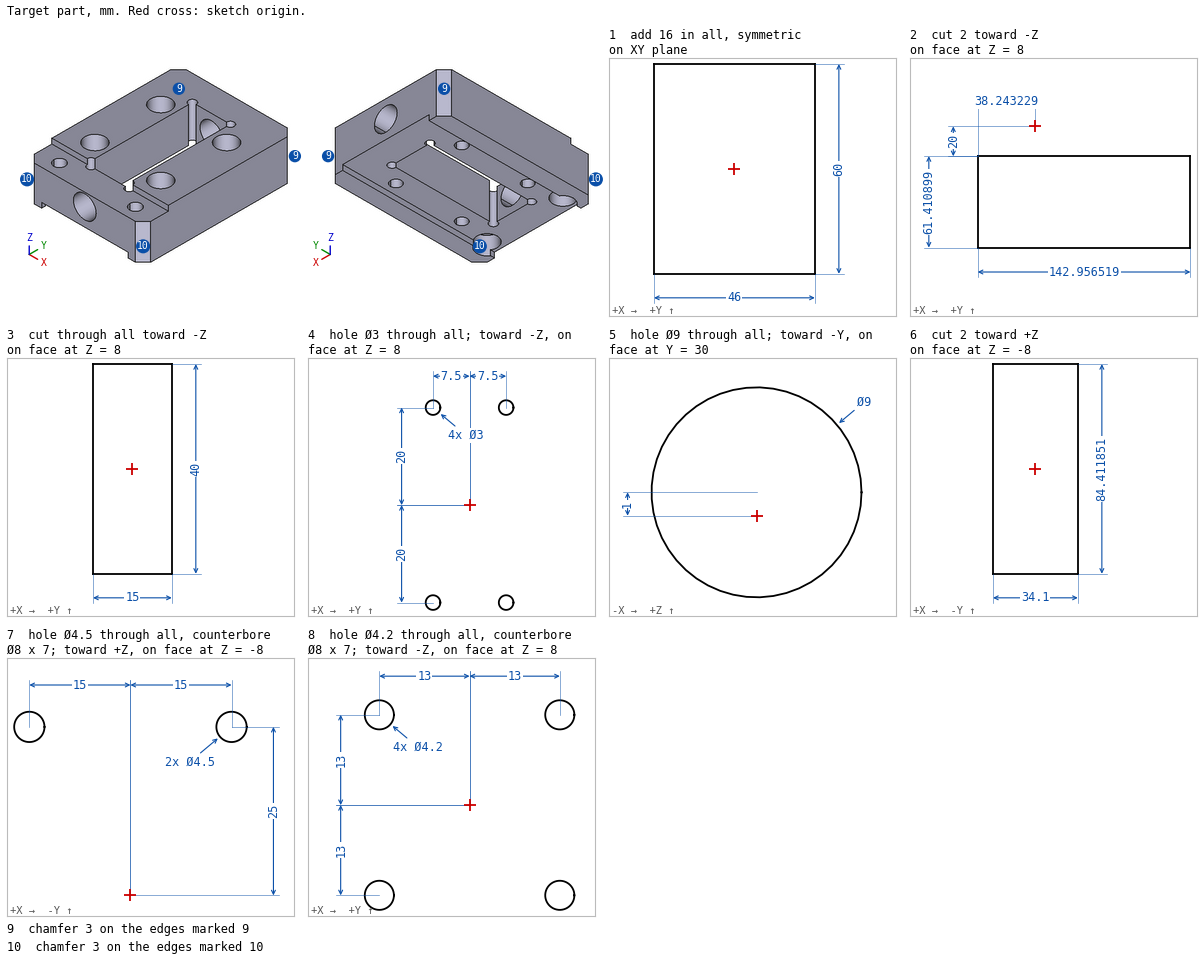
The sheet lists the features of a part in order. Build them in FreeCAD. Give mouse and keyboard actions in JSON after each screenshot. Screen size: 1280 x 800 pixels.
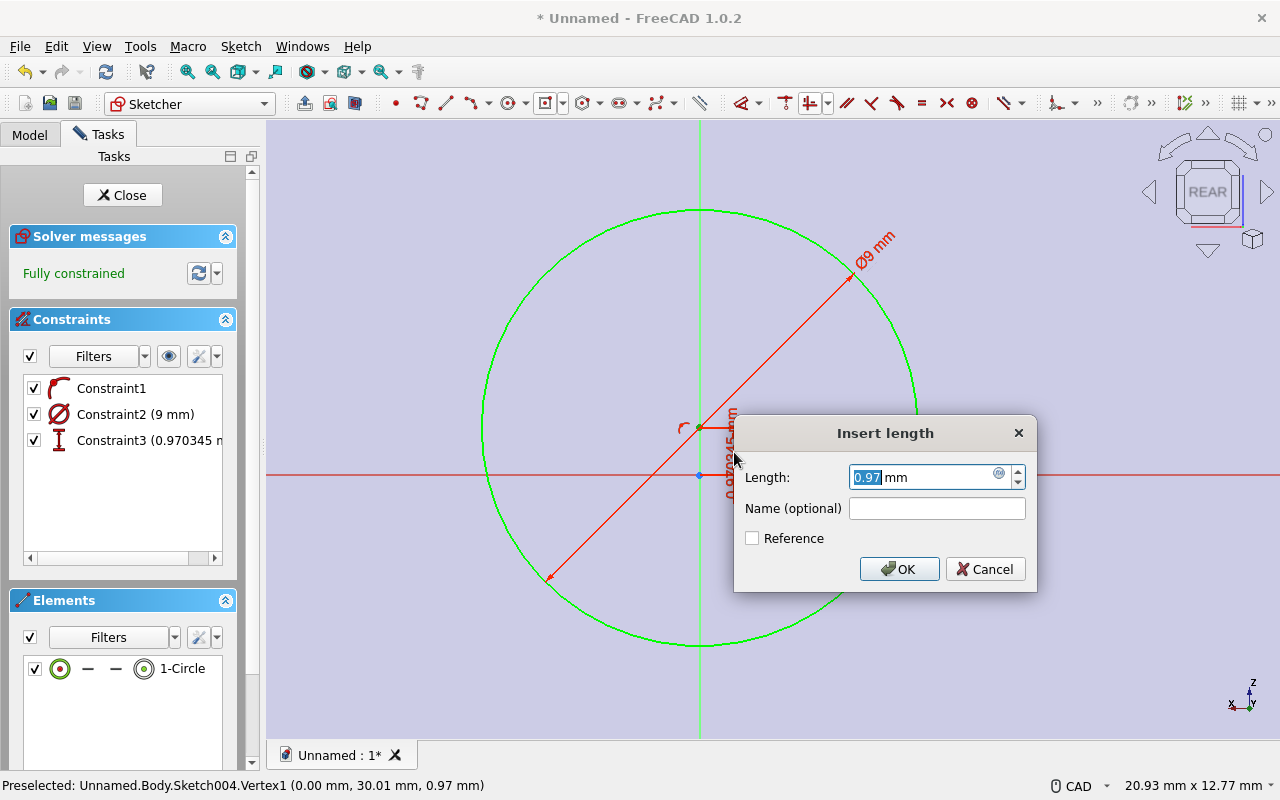
{"action": "type", "text": "1"}
{"action": "key", "text": "Return"}
{"action": "key", "text": "Escape"}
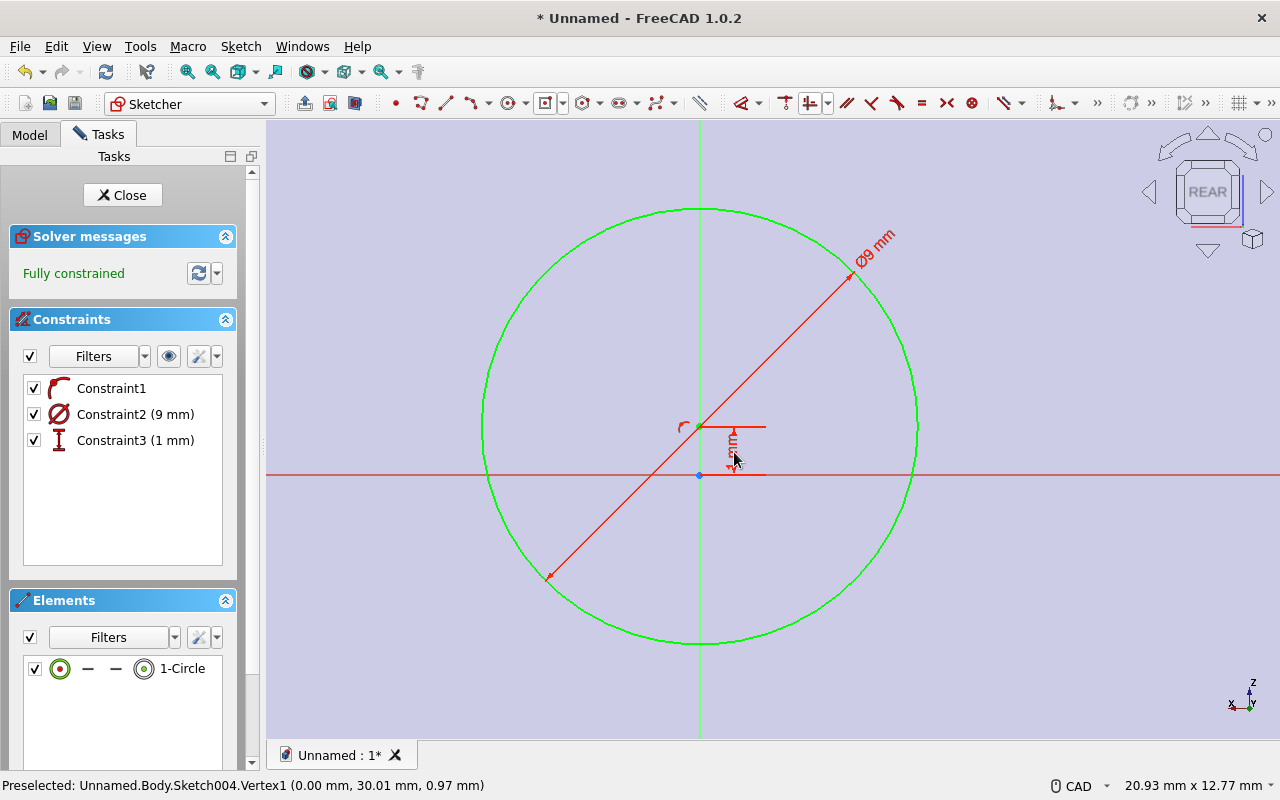
{"action": "left_click", "coordinate": [123, 195]}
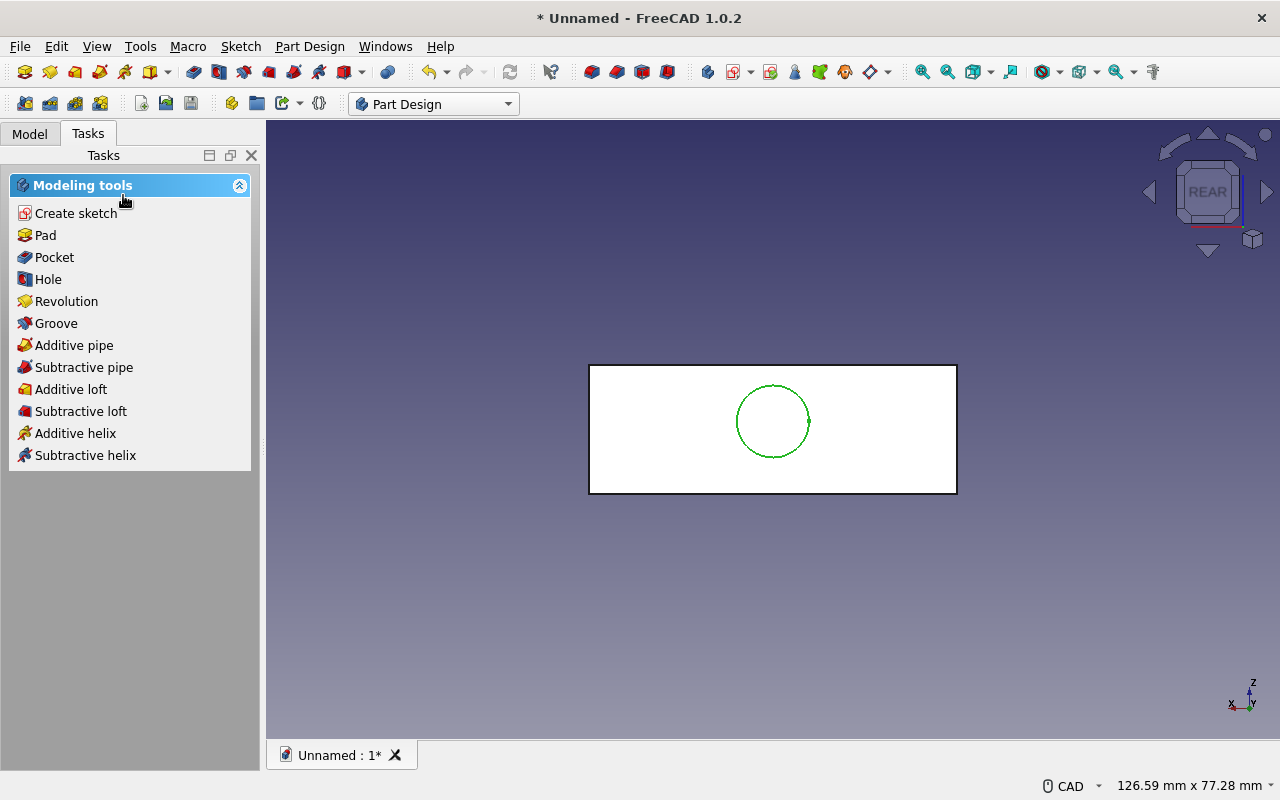
{"action": "left_click", "coordinate": [219, 72]}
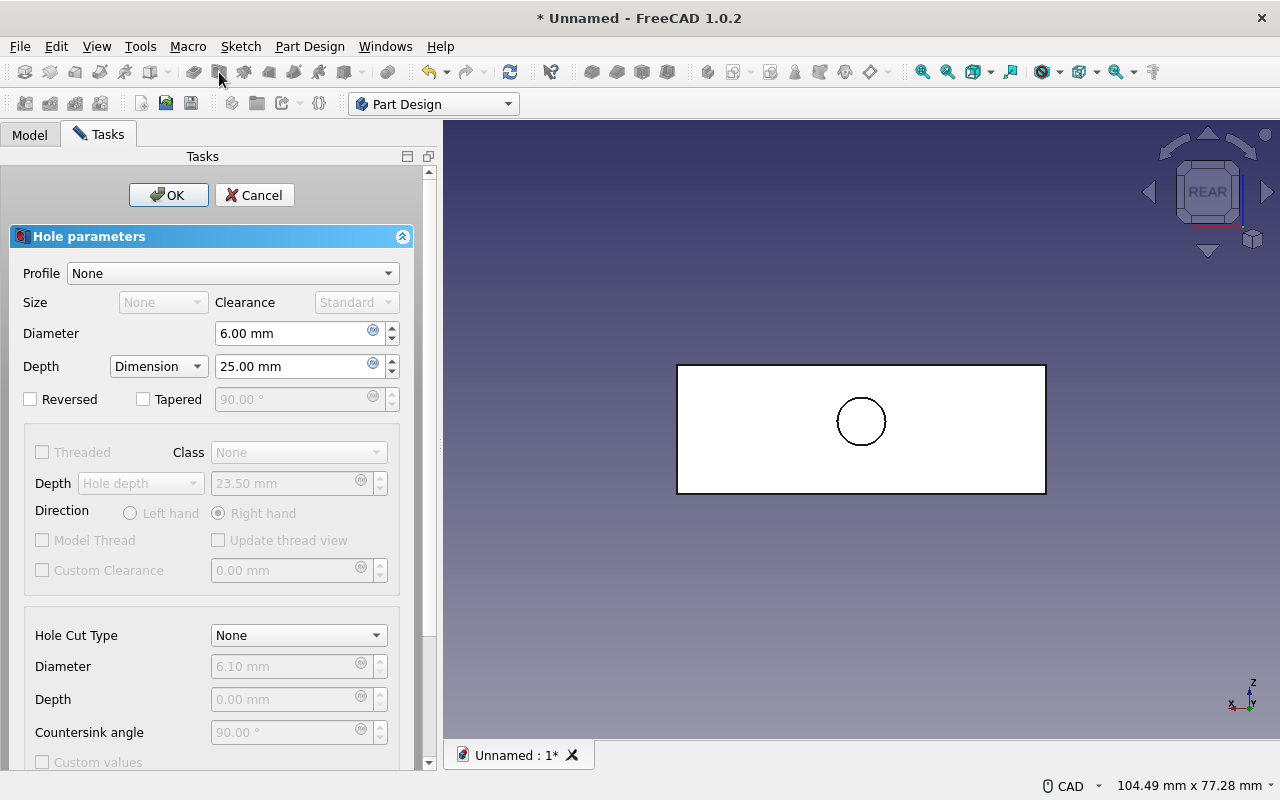
{"action": "triple_click", "coordinate": [300, 334]}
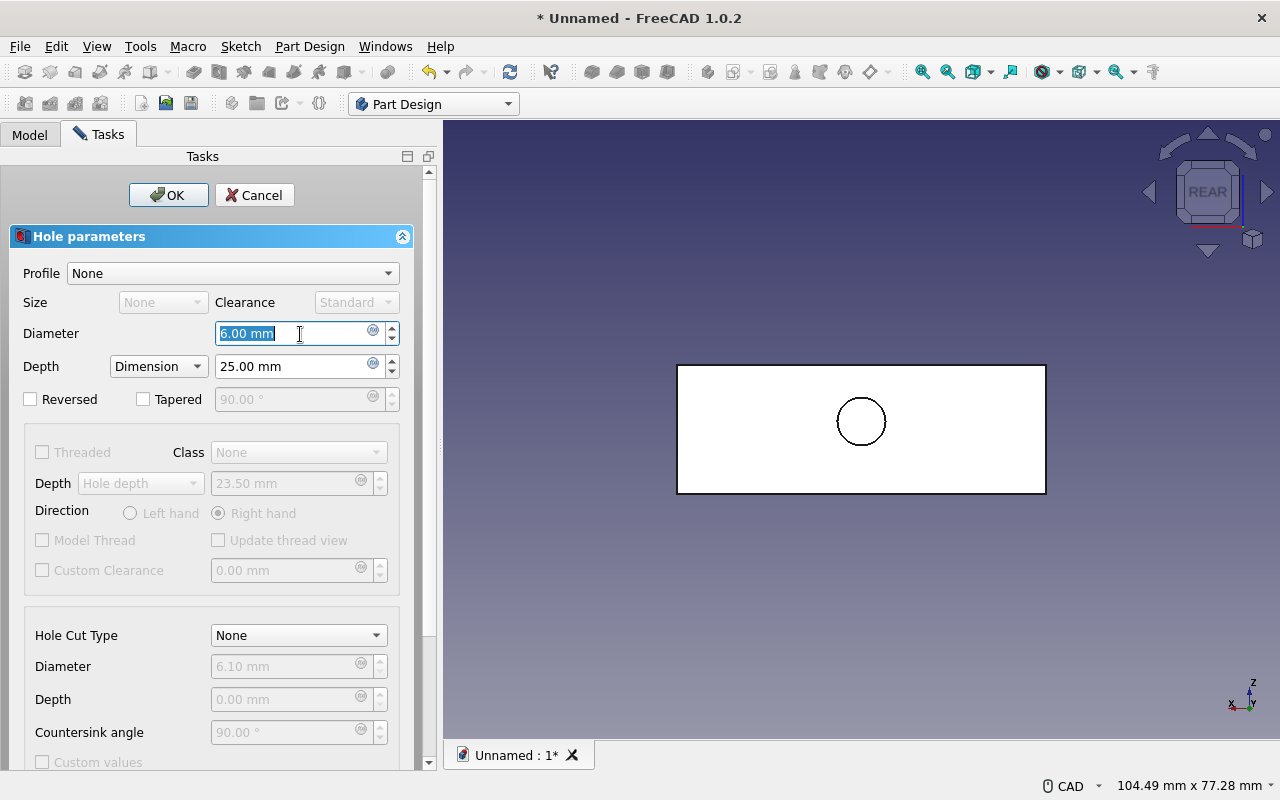
{"action": "type", "text": "9"}
{"action": "key", "text": "Tab"}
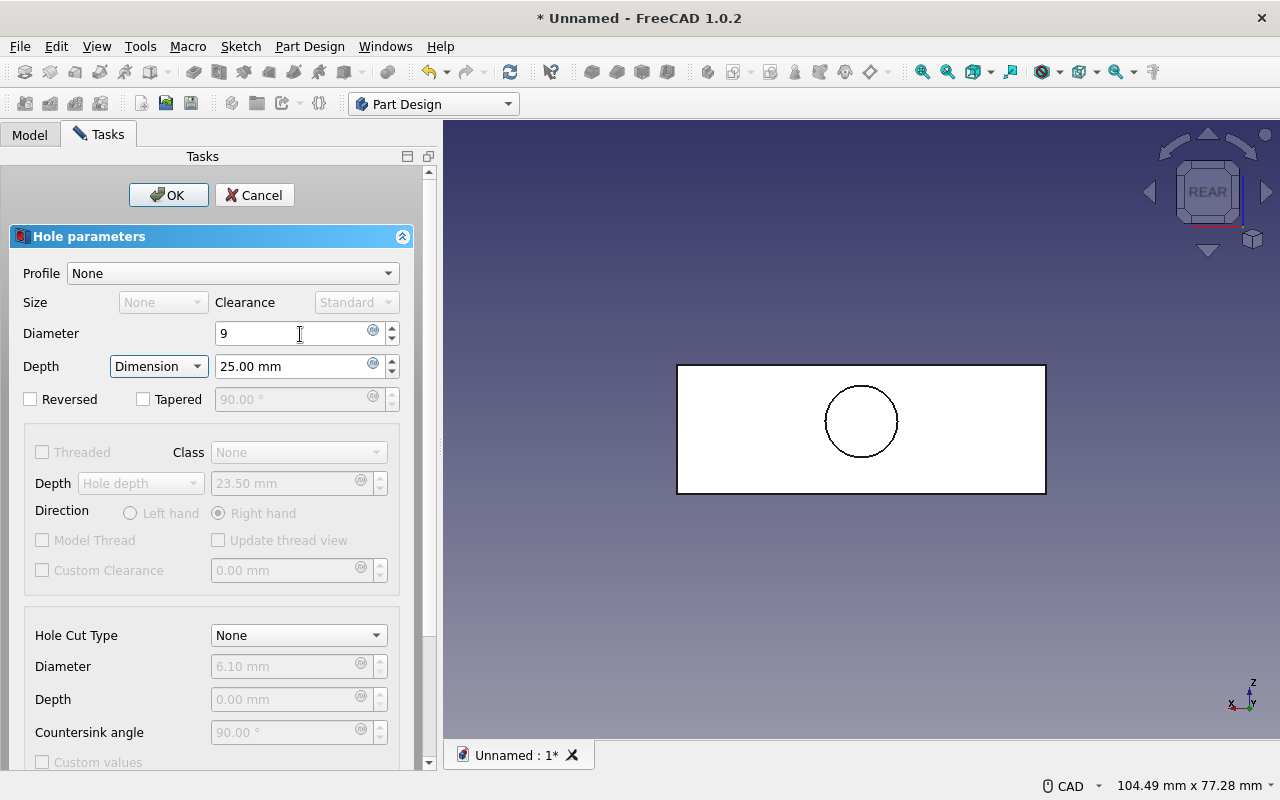
{"action": "left_click", "coordinate": [160, 366]}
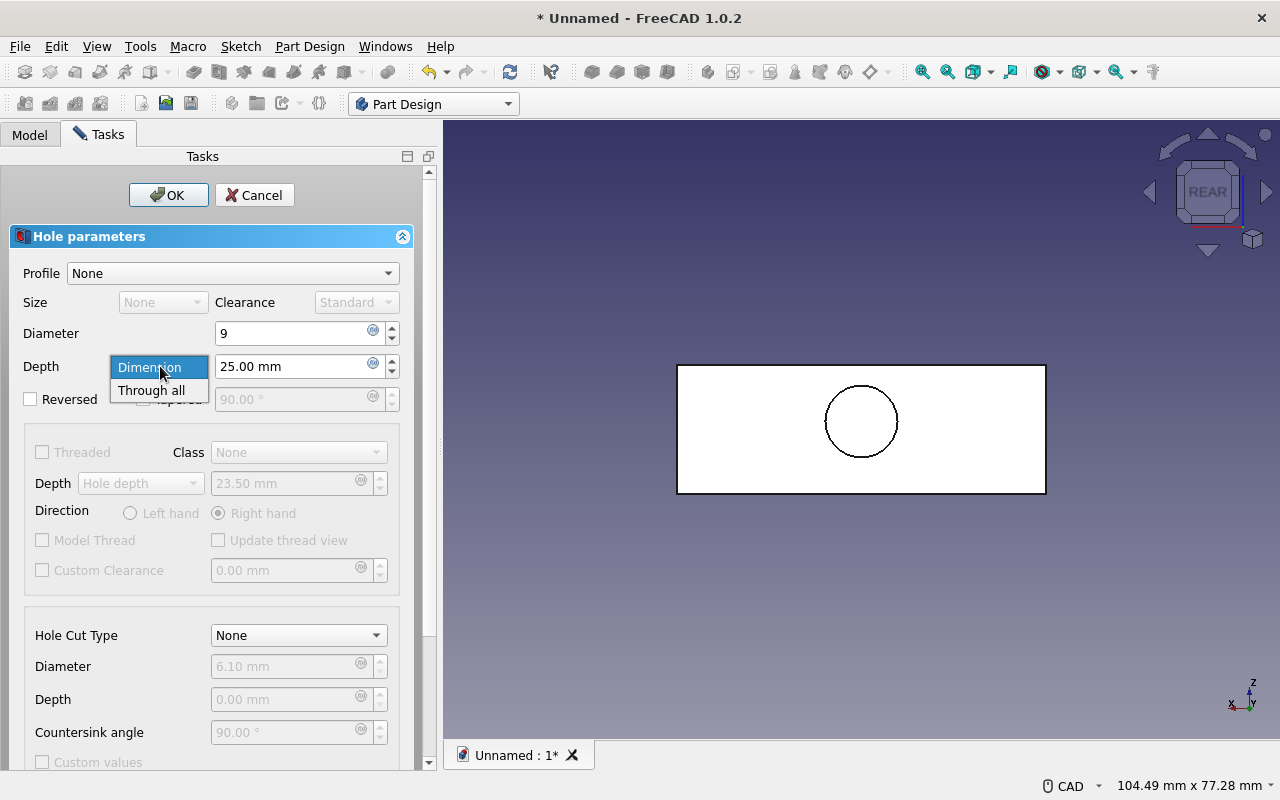
{"action": "left_click", "coordinate": [158, 390]}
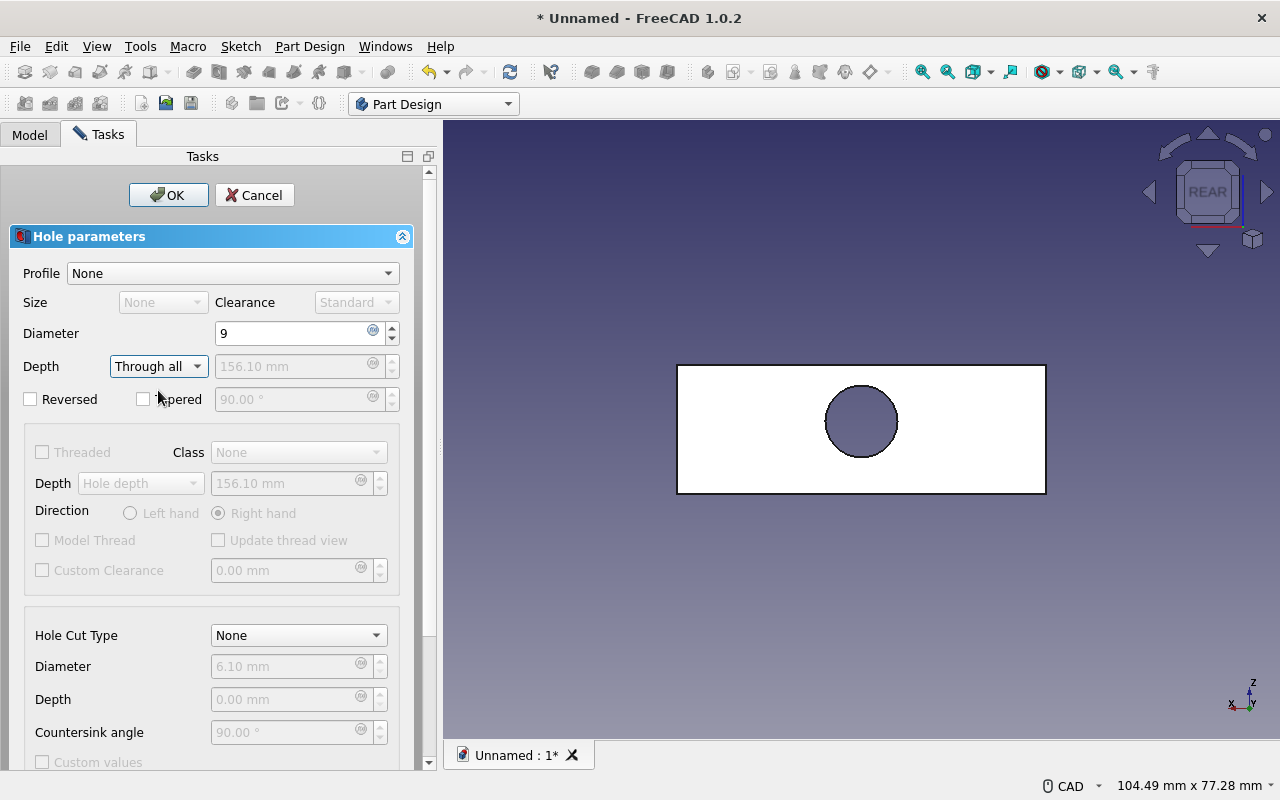
{"action": "left_click", "coordinate": [169, 195]}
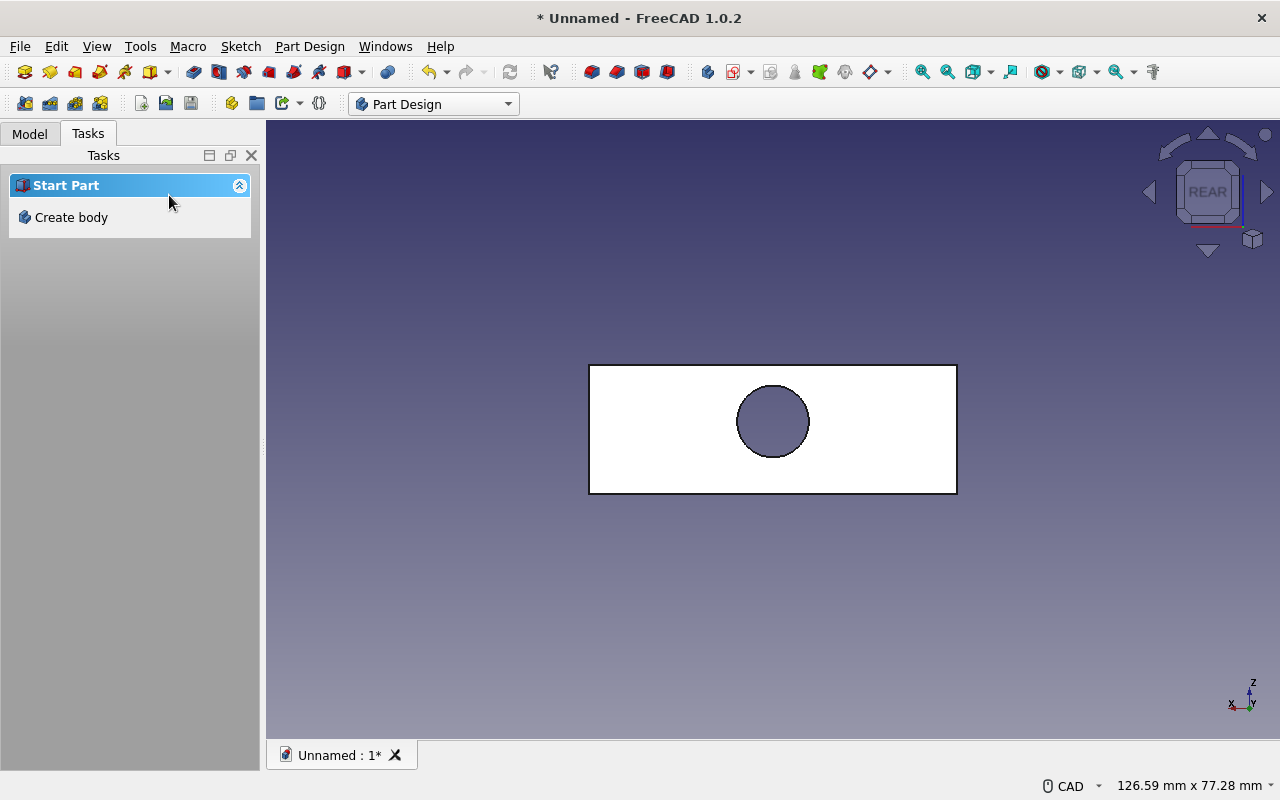
{"action": "left_click", "coordinate": [923, 72]}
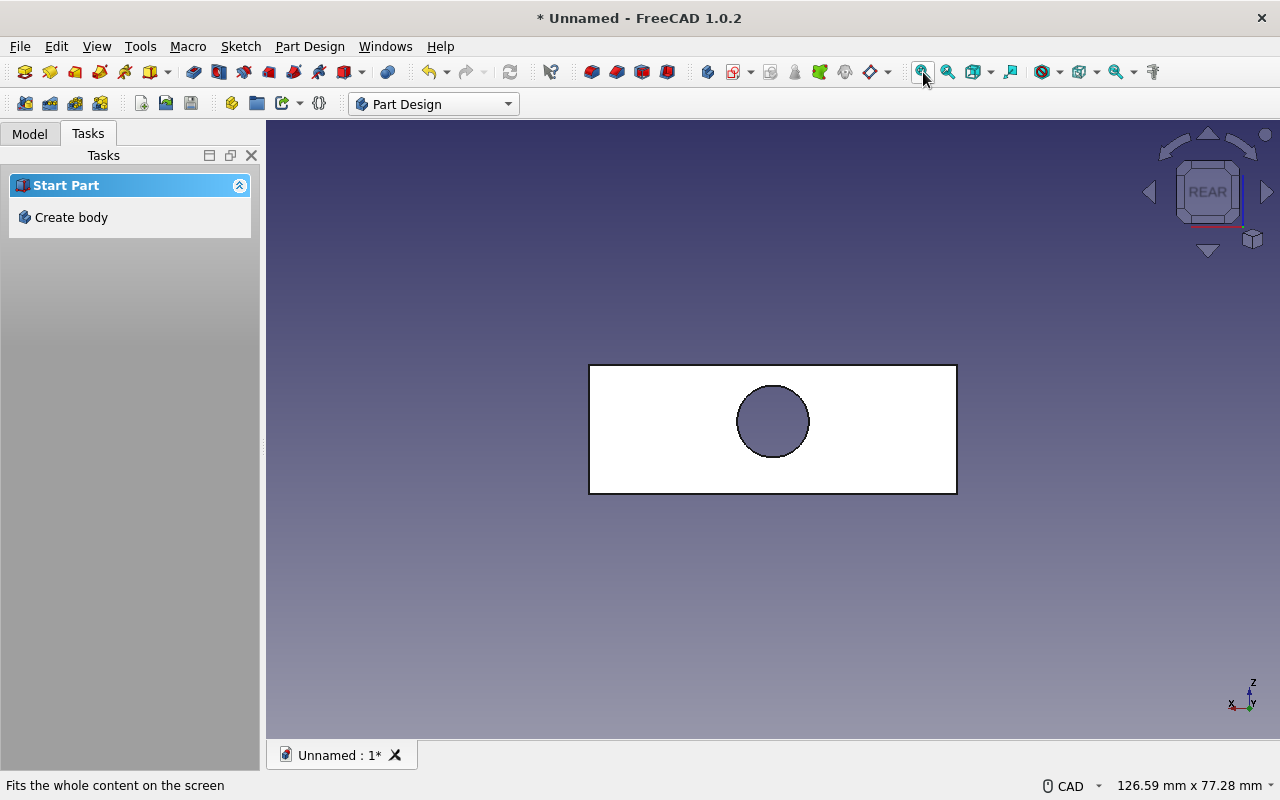
{"action": "key", "text": "5"}